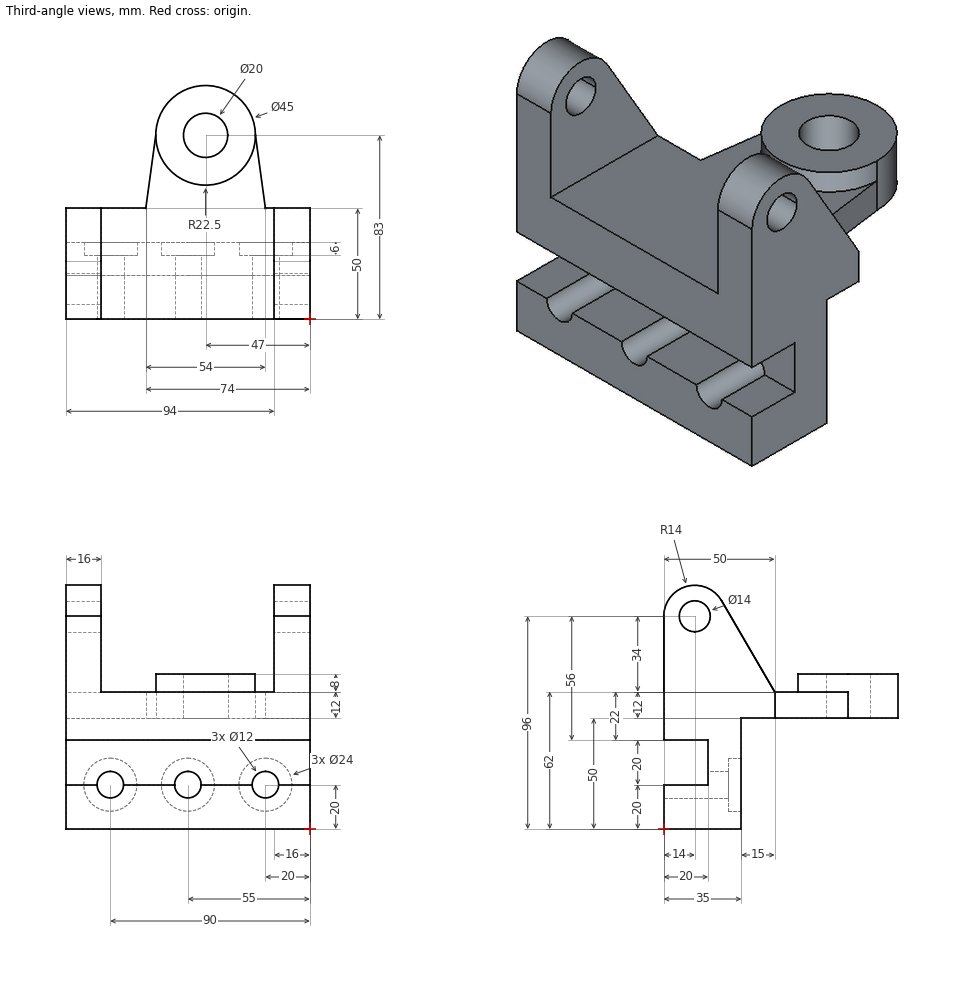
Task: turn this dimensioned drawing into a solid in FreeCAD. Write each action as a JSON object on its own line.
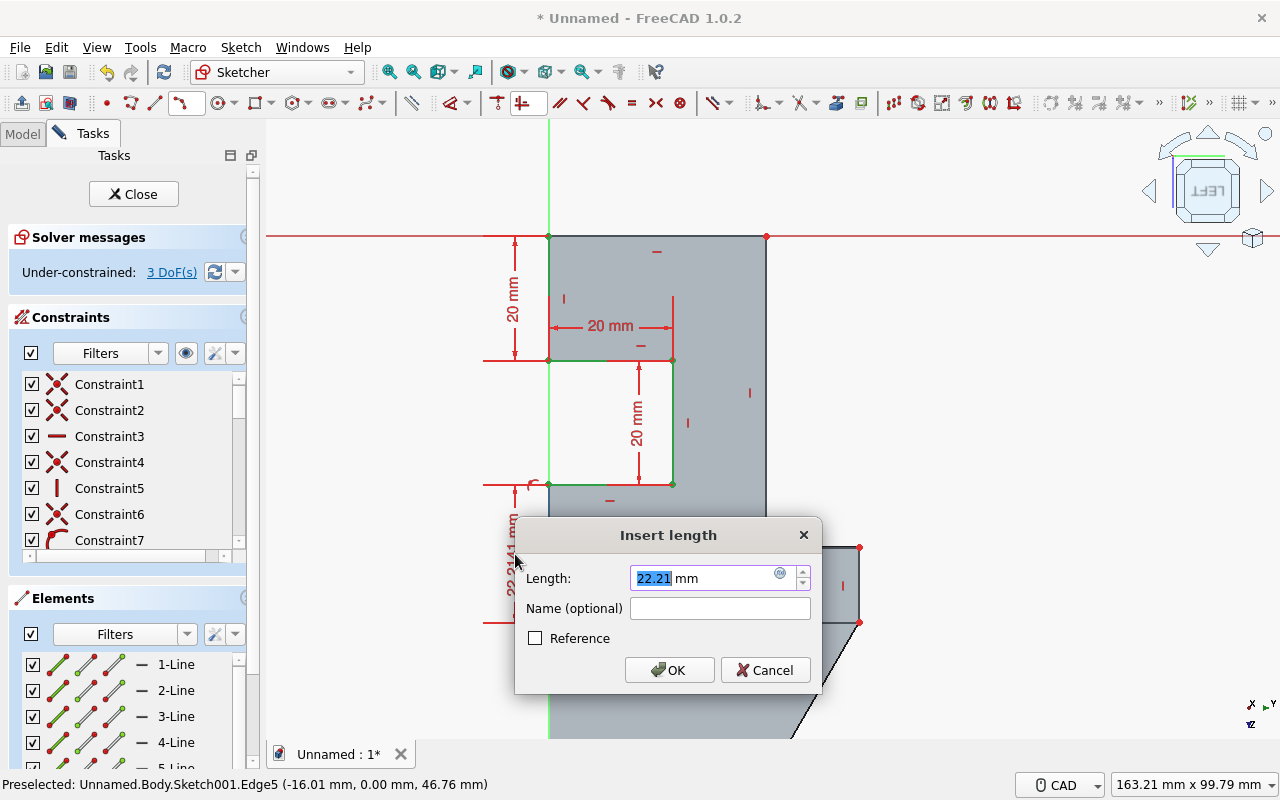
{"action": "type", "text": "22"}
{"action": "key", "text": "Return"}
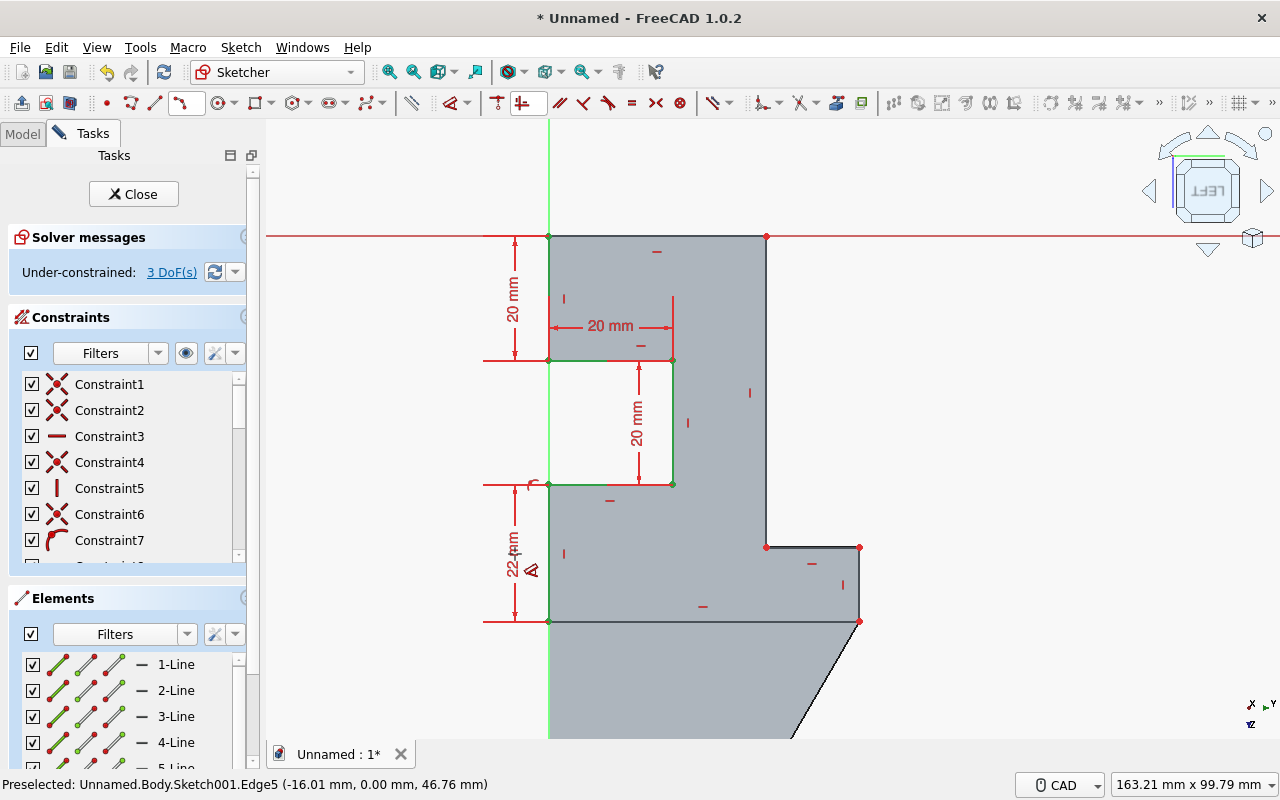
{"action": "left_click", "coordinate": [642, 622]}
{"action": "left_click", "coordinate": [704, 656]}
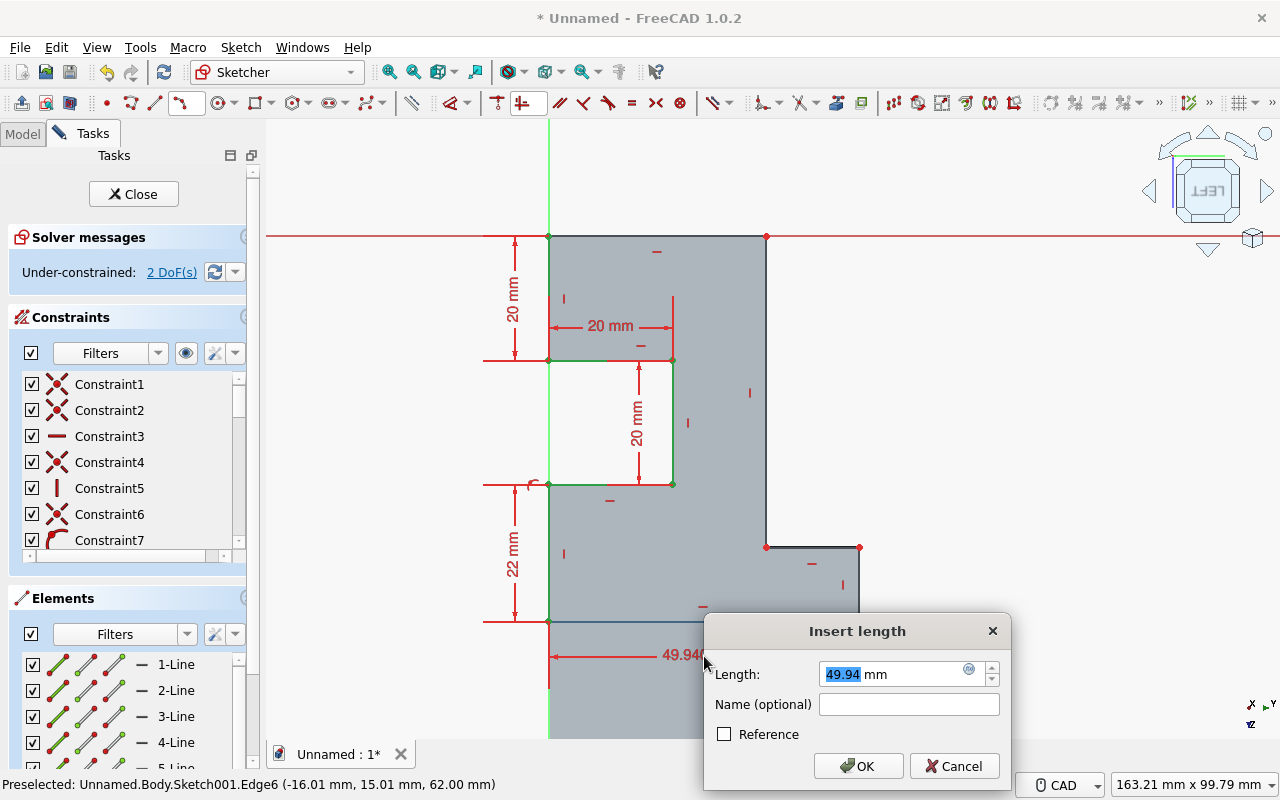
{"action": "type", "text": "50"}
{"action": "key", "text": "Return"}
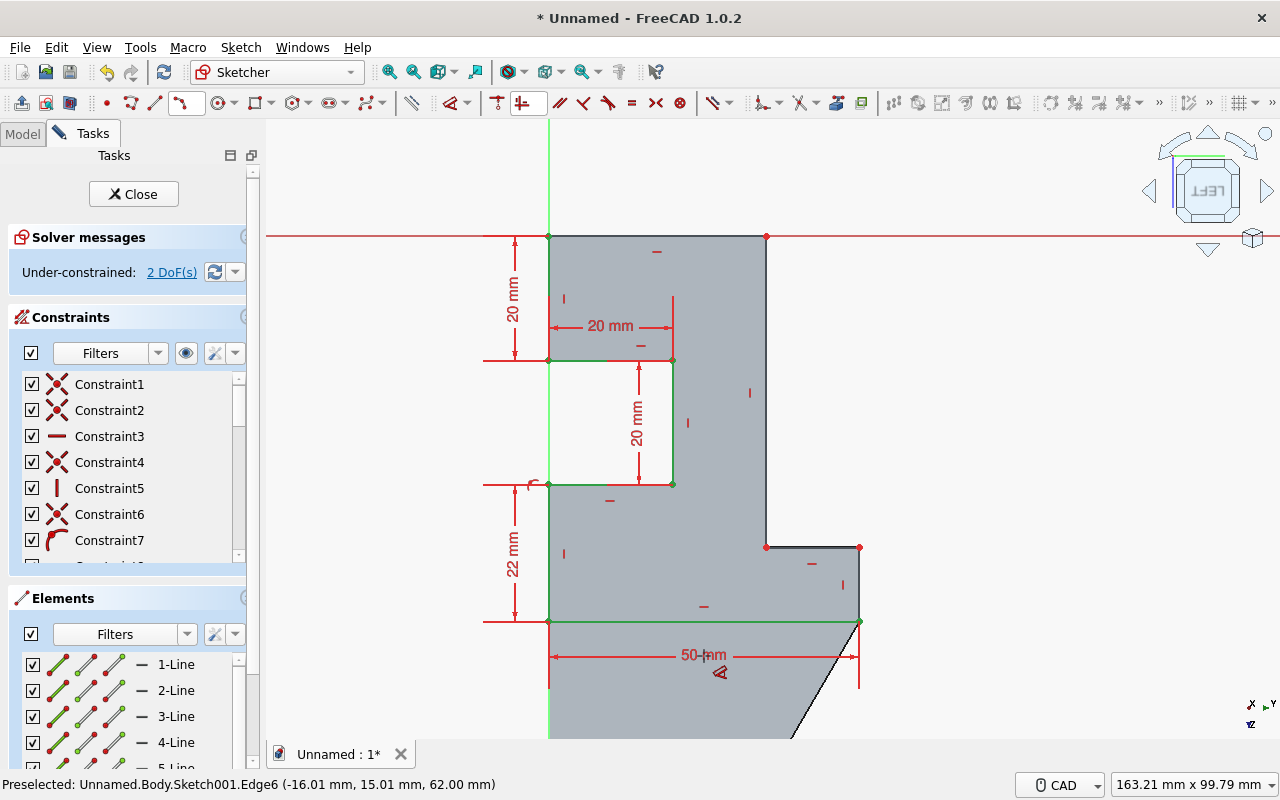
{"action": "left_click", "coordinate": [859, 600]}
{"action": "left_click", "coordinate": [893, 585]}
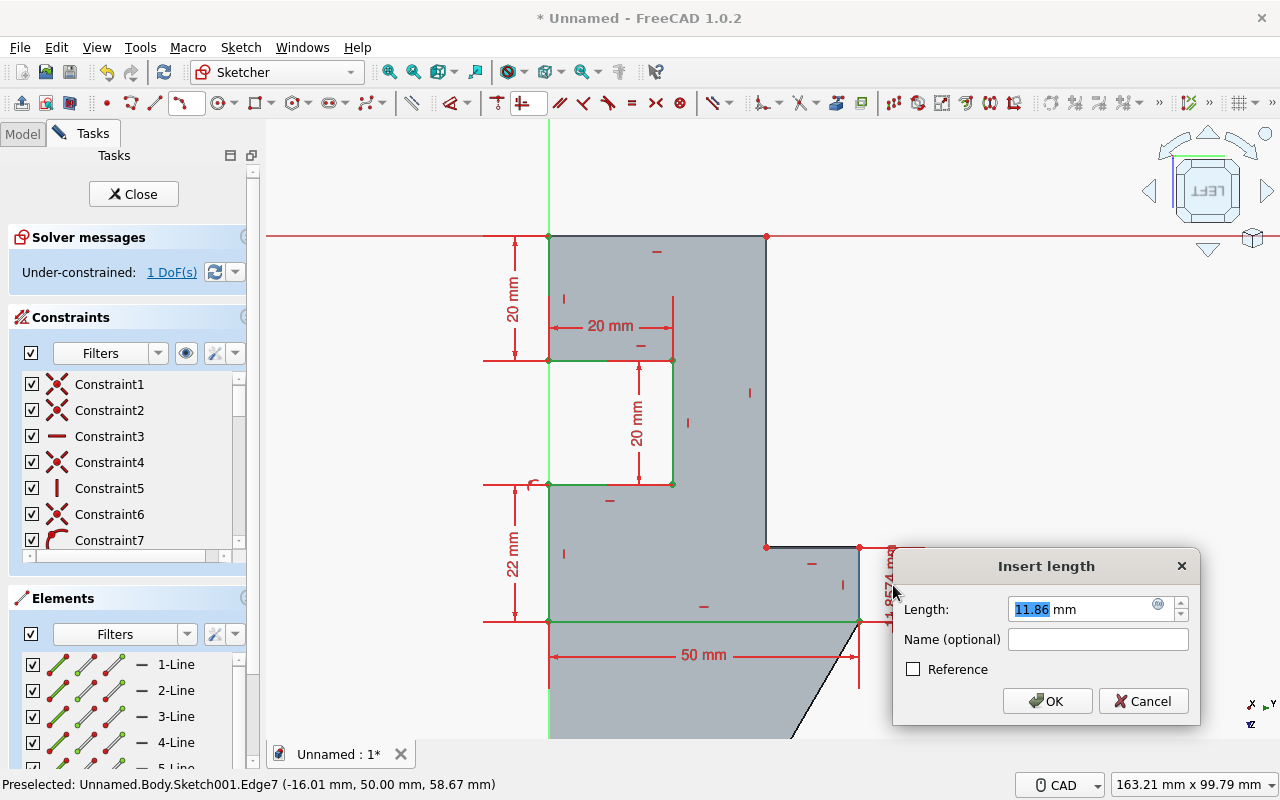
{"action": "type", "text": "12"}
{"action": "key", "text": "Return"}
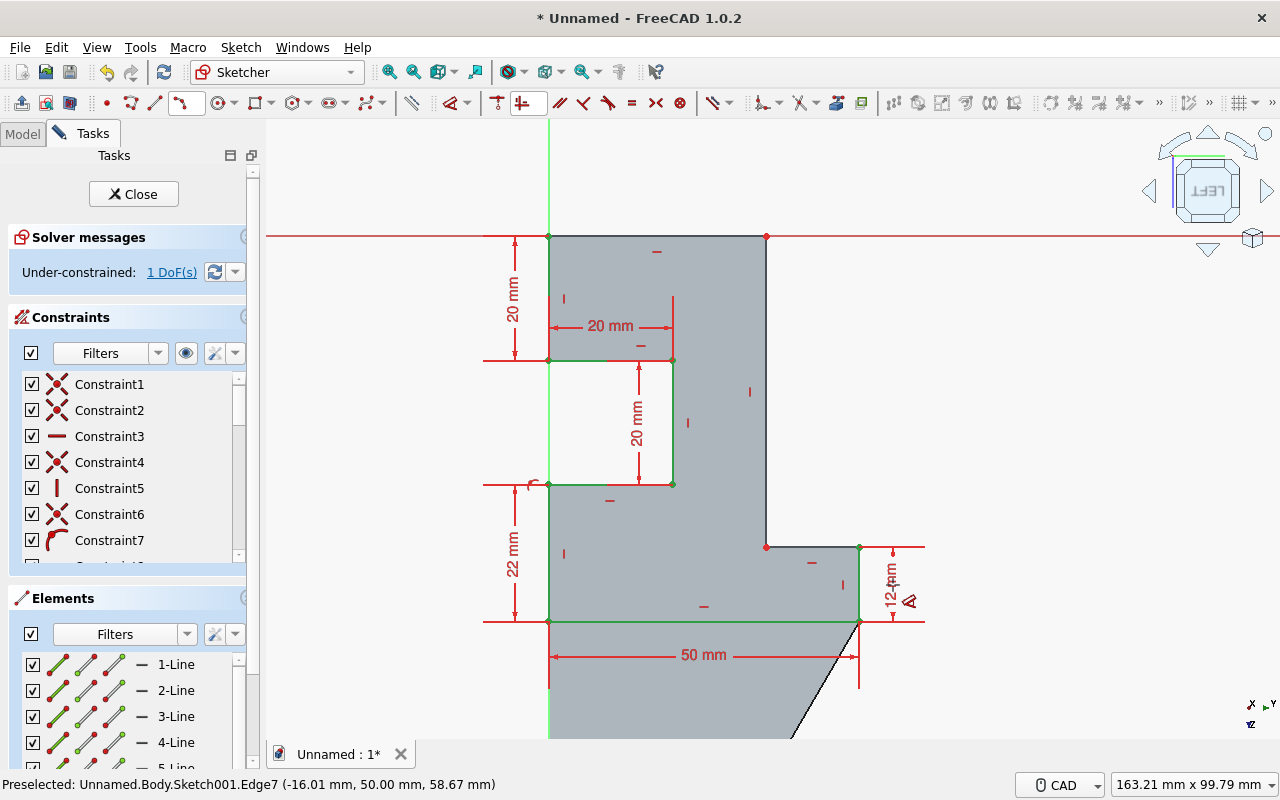
{"action": "left_click", "coordinate": [831, 547]}
{"action": "left_click", "coordinate": [813, 581]}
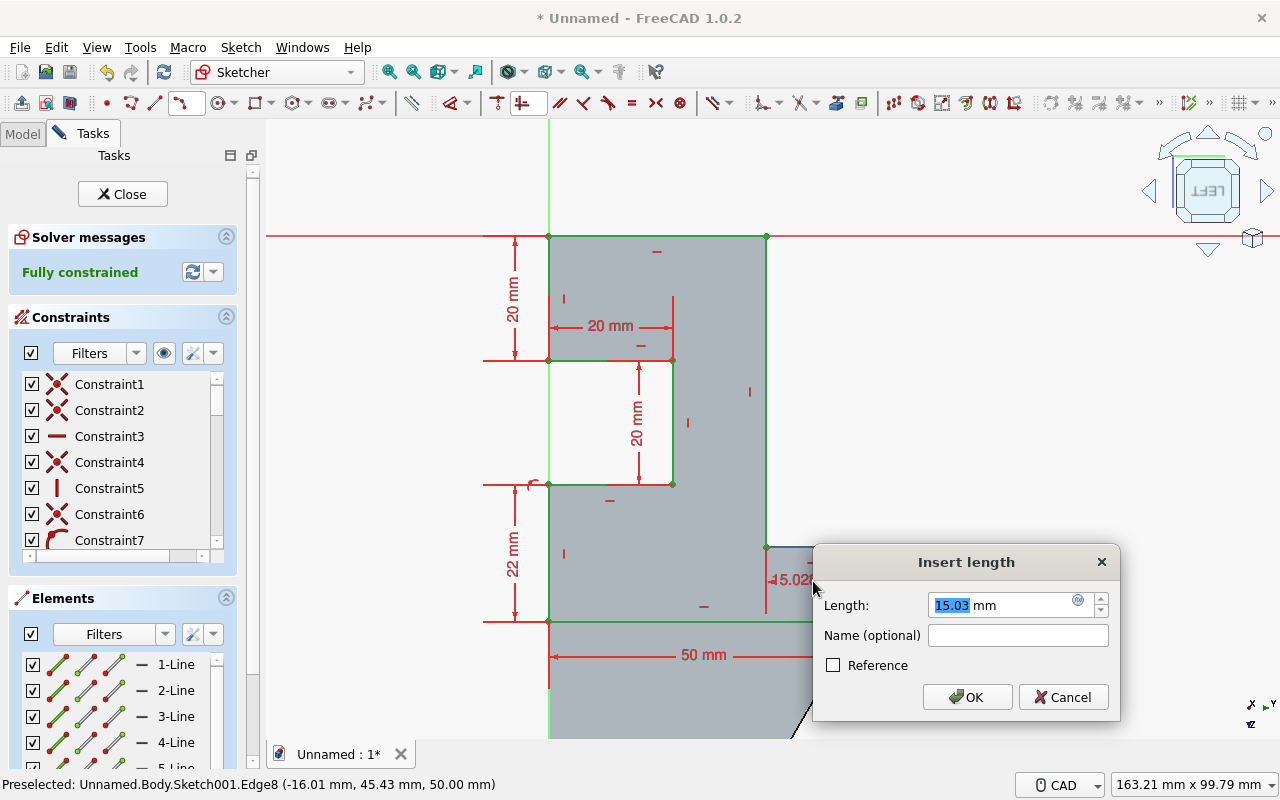
{"action": "type", "text": "15"}
{"action": "key", "text": "Return"}
{"action": "key", "text": "Escape"}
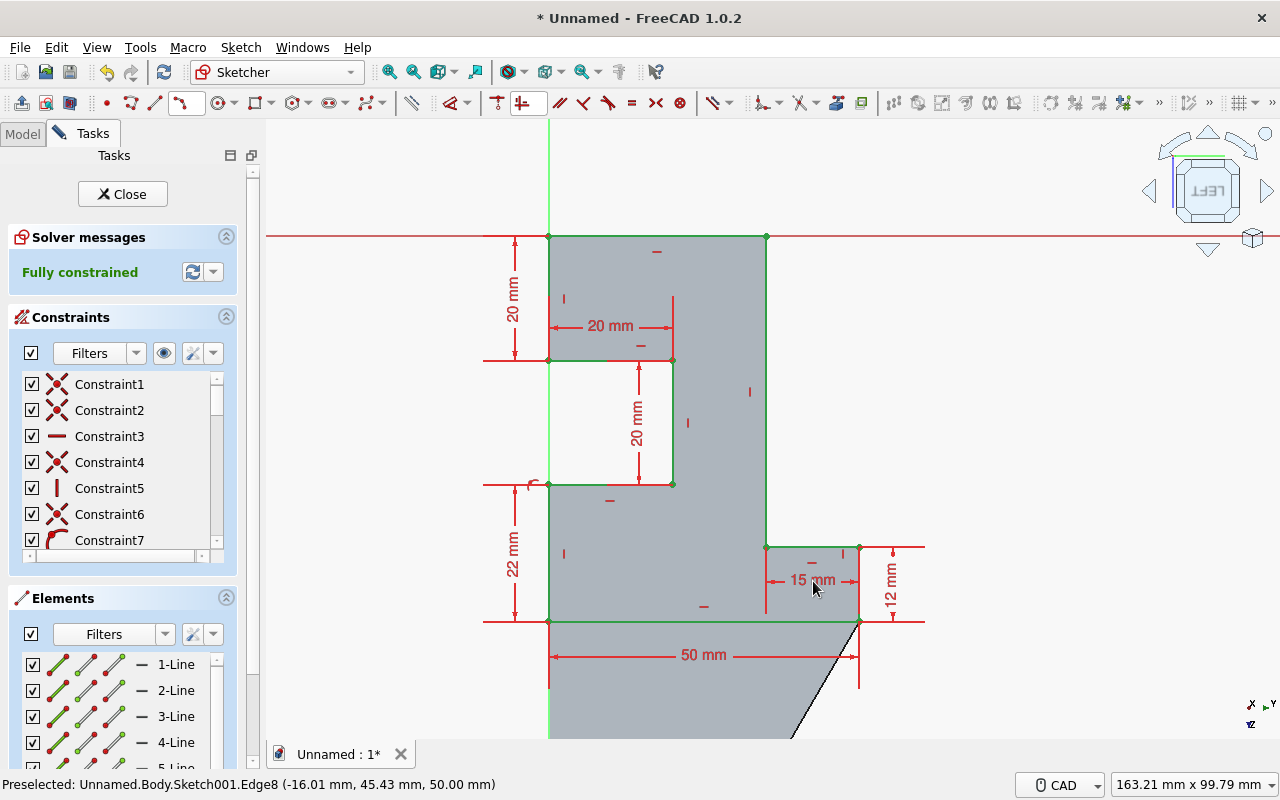
{"action": "left_click", "coordinate": [123, 194]}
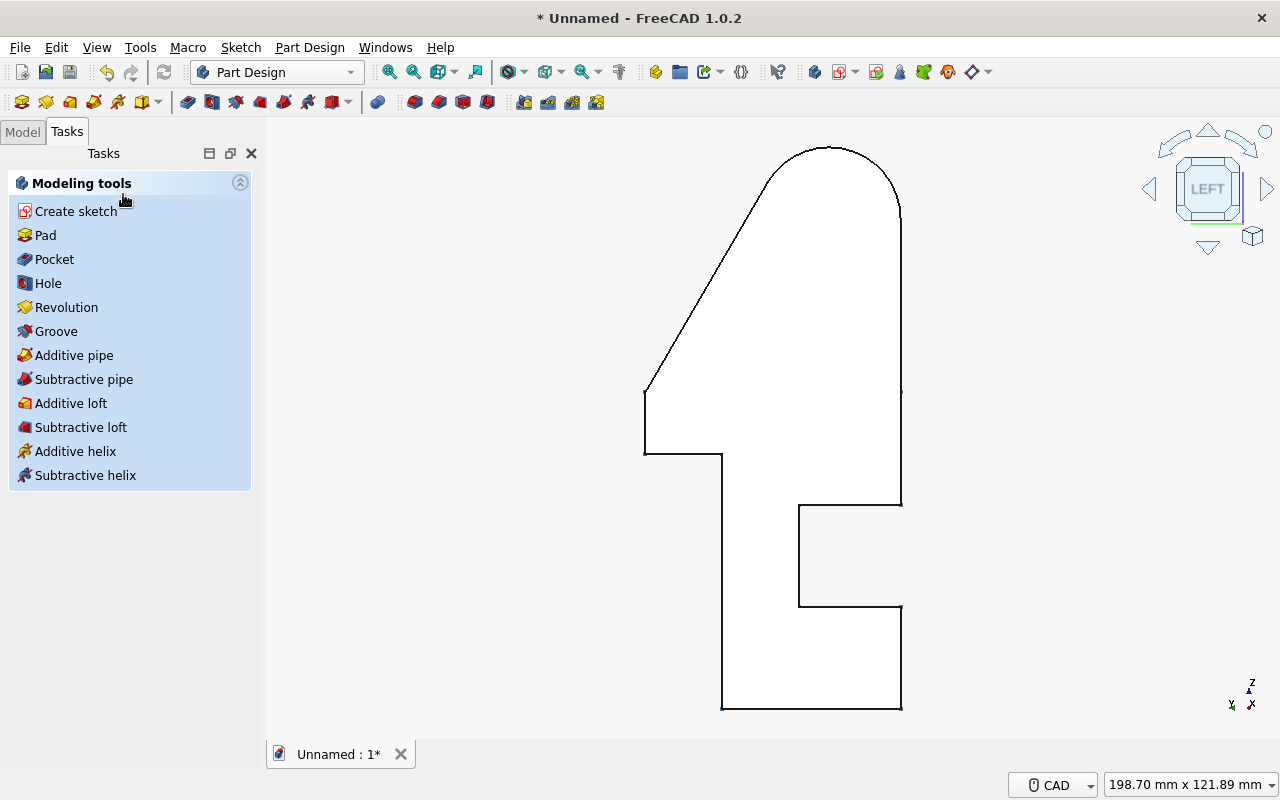
{"action": "left_click", "coordinate": [22, 102]}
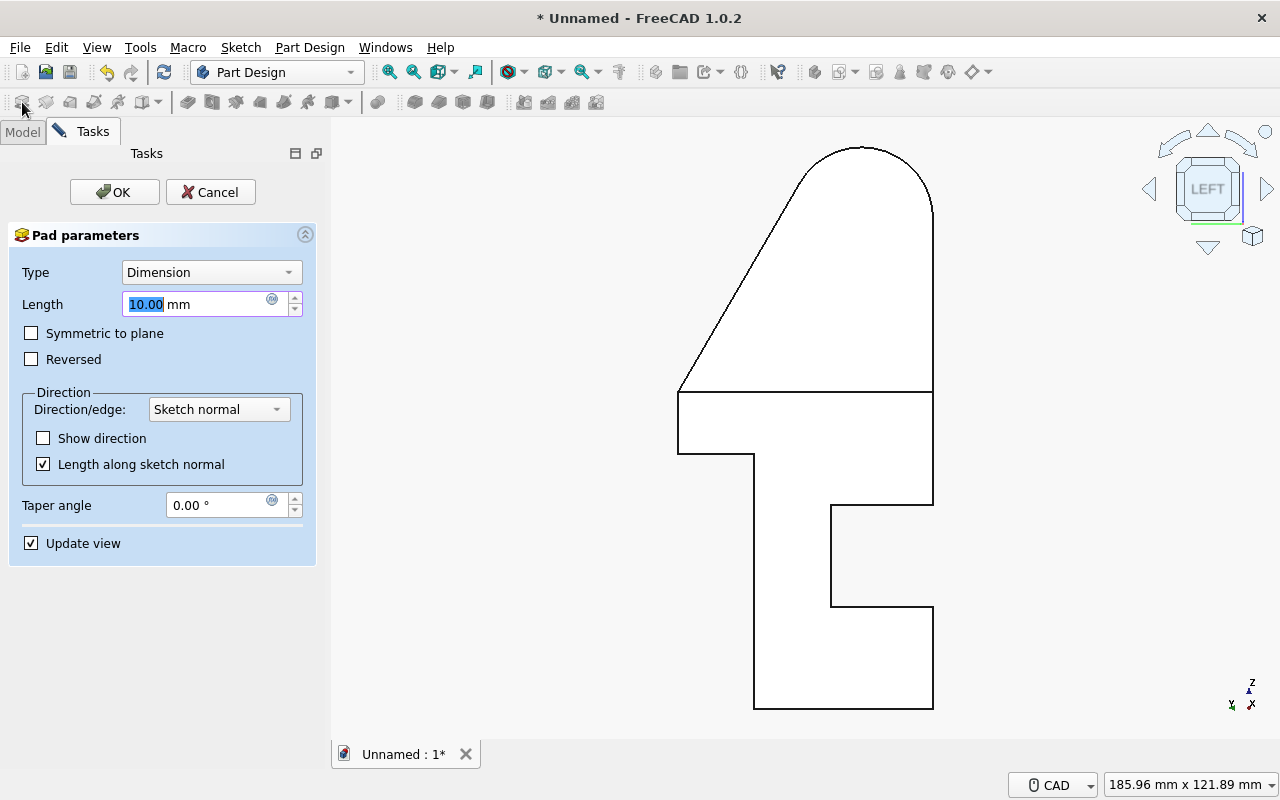
{"action": "type", "text": "94"}
{"action": "key", "text": "Tab"}